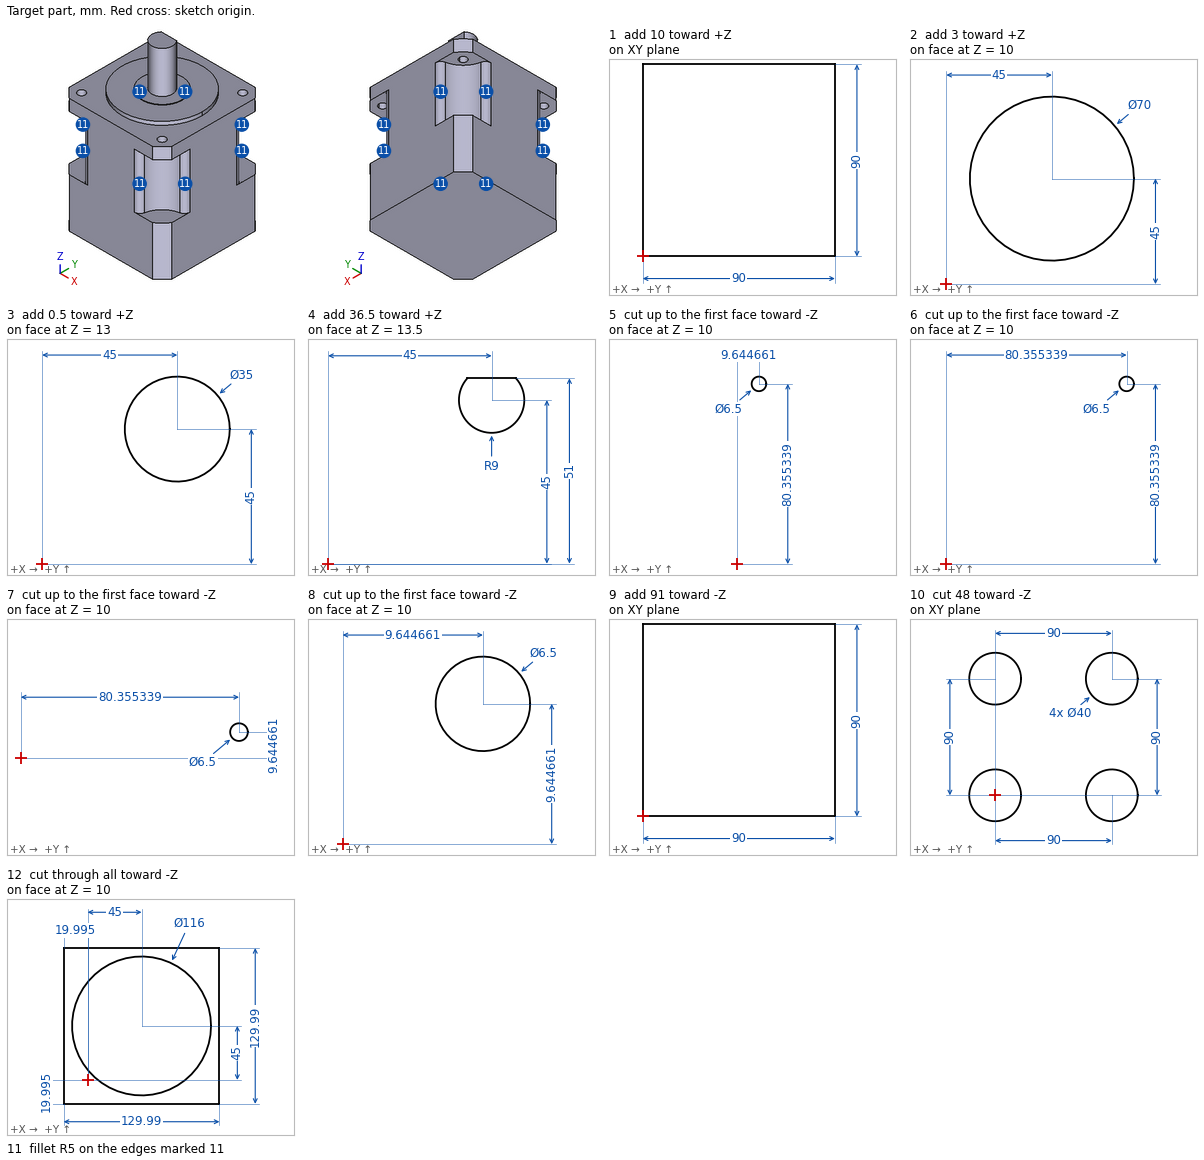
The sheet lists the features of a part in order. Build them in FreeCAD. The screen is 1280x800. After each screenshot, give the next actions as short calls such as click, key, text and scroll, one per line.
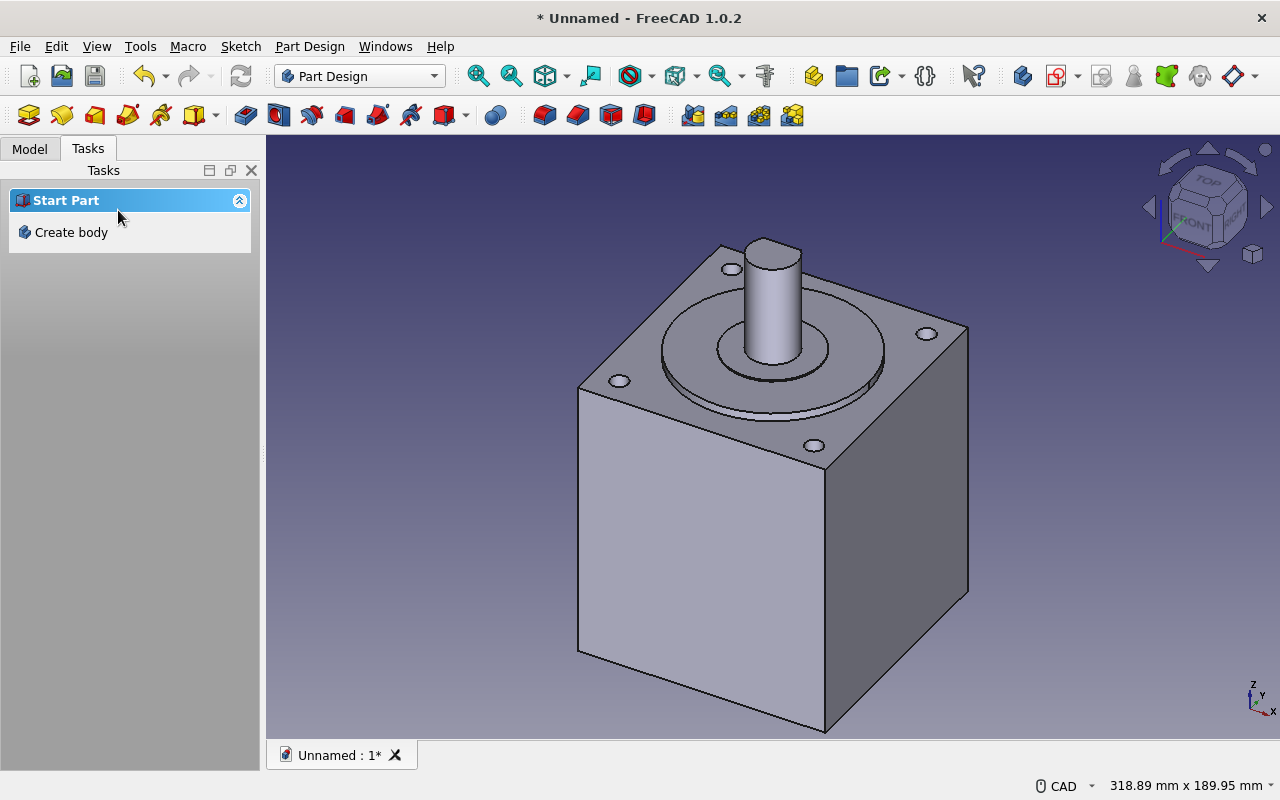
click(1056, 76)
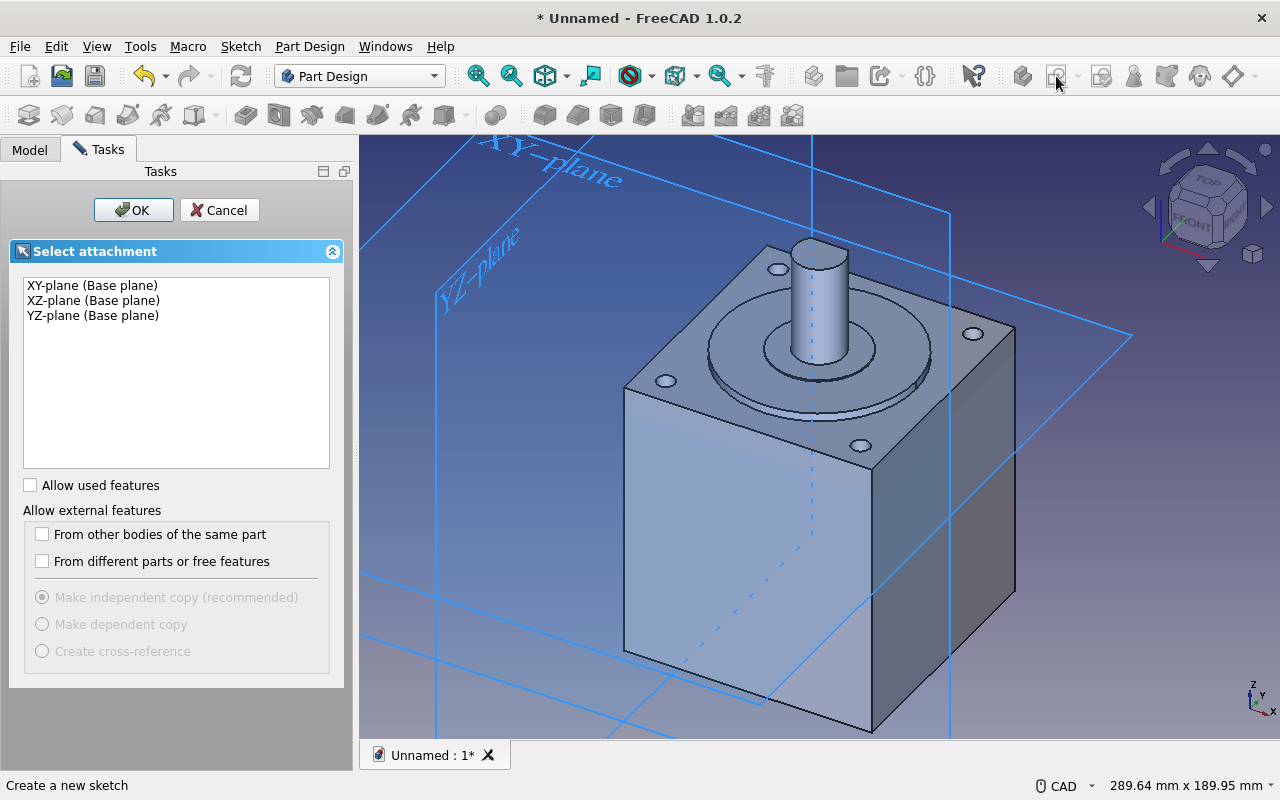
click(84, 286)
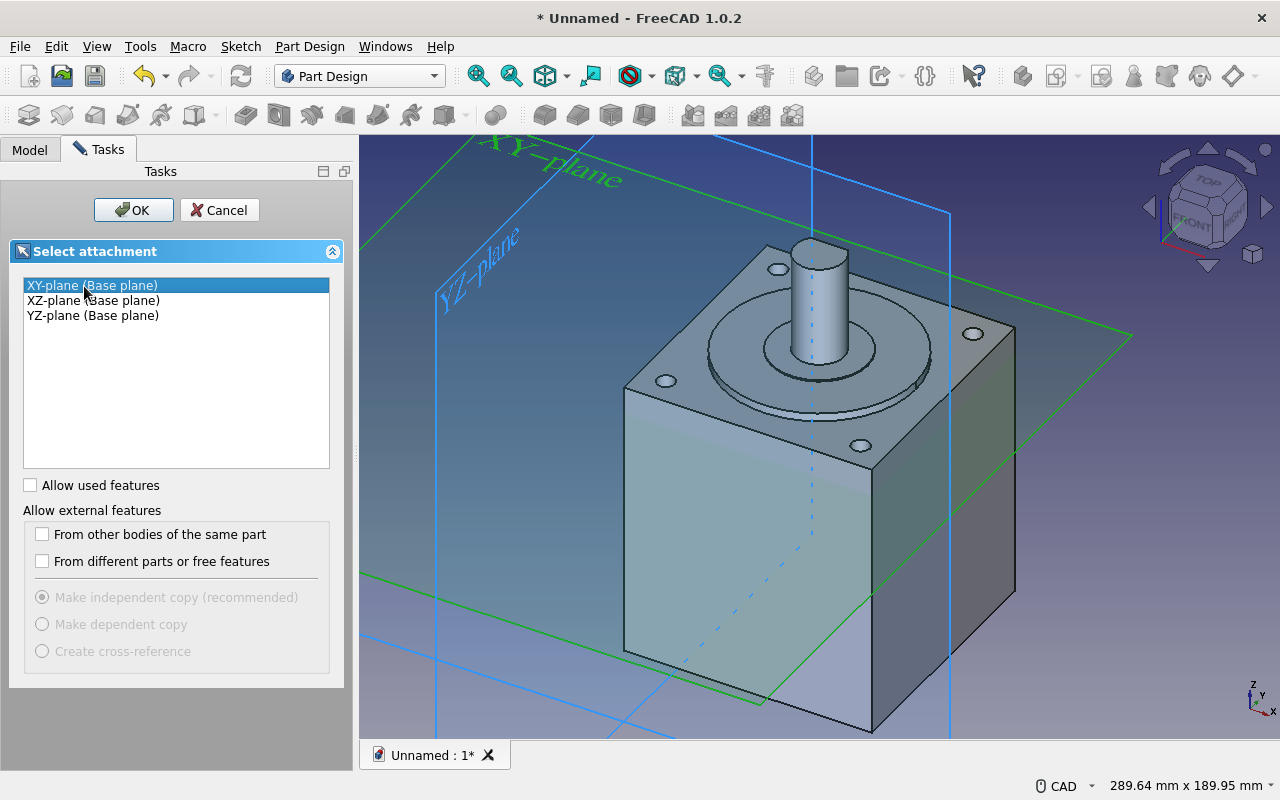
click(134, 210)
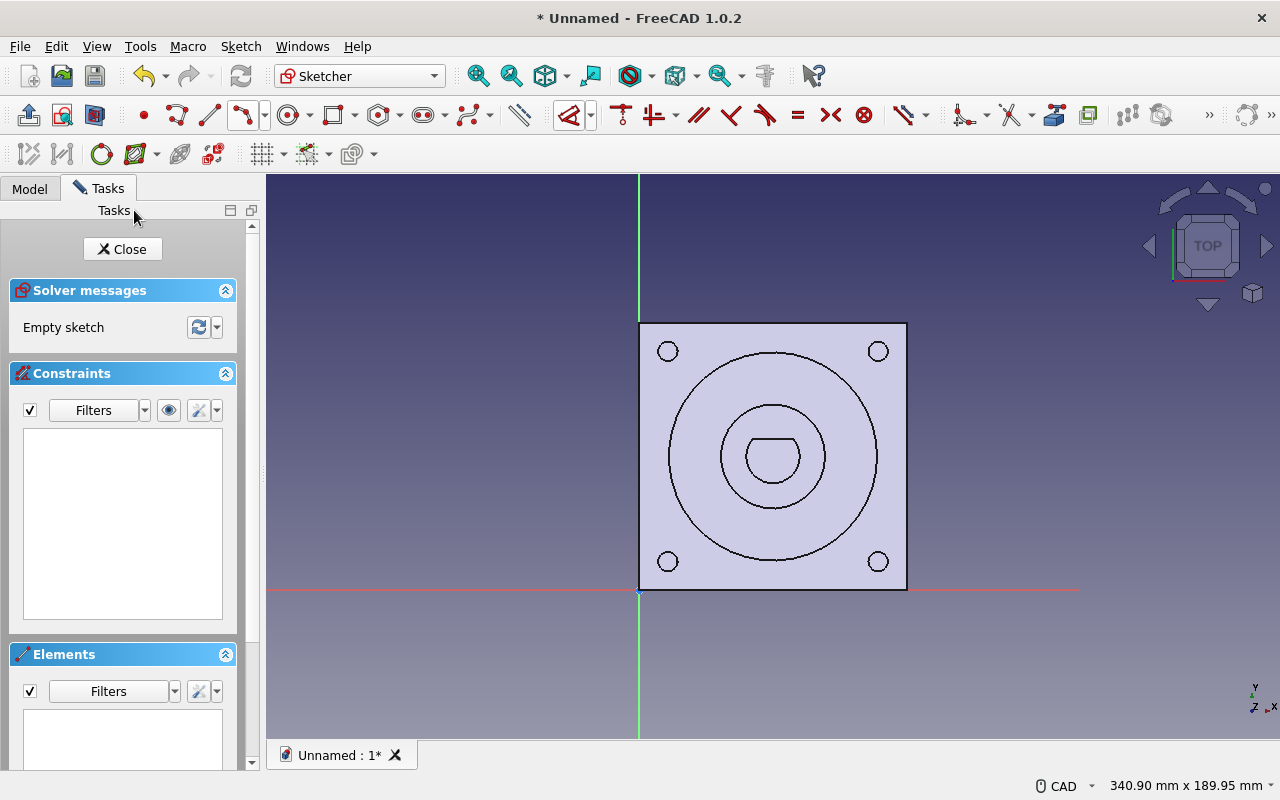
key(q)
key(s)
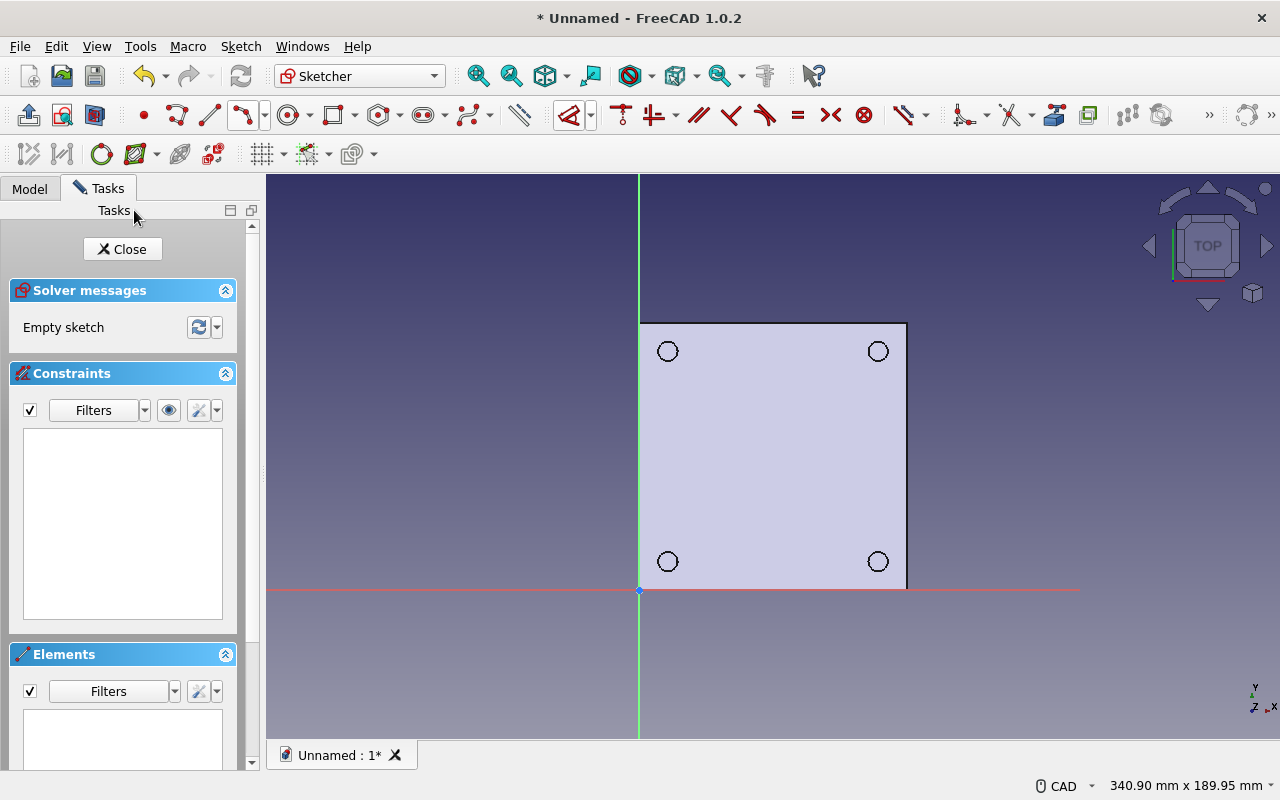
key(g)
key(c)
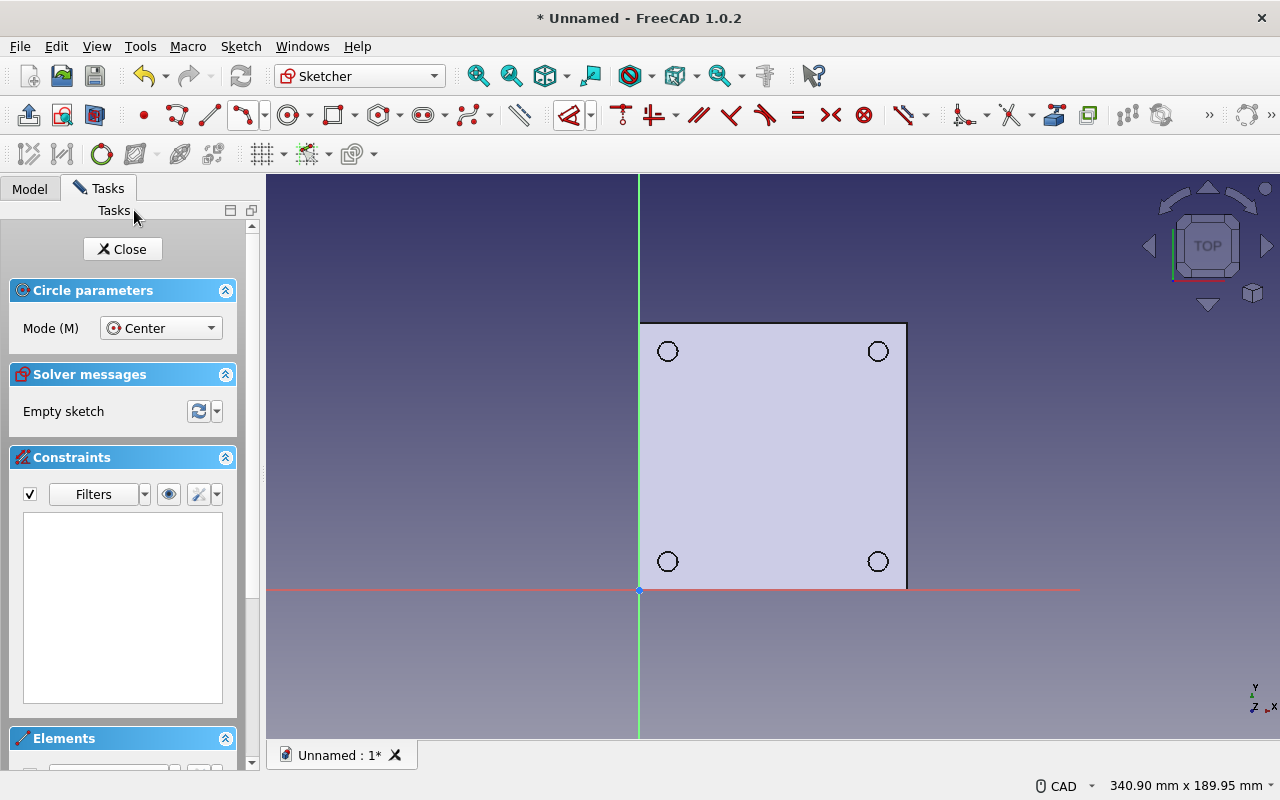
click(907, 323)
move(949, 281)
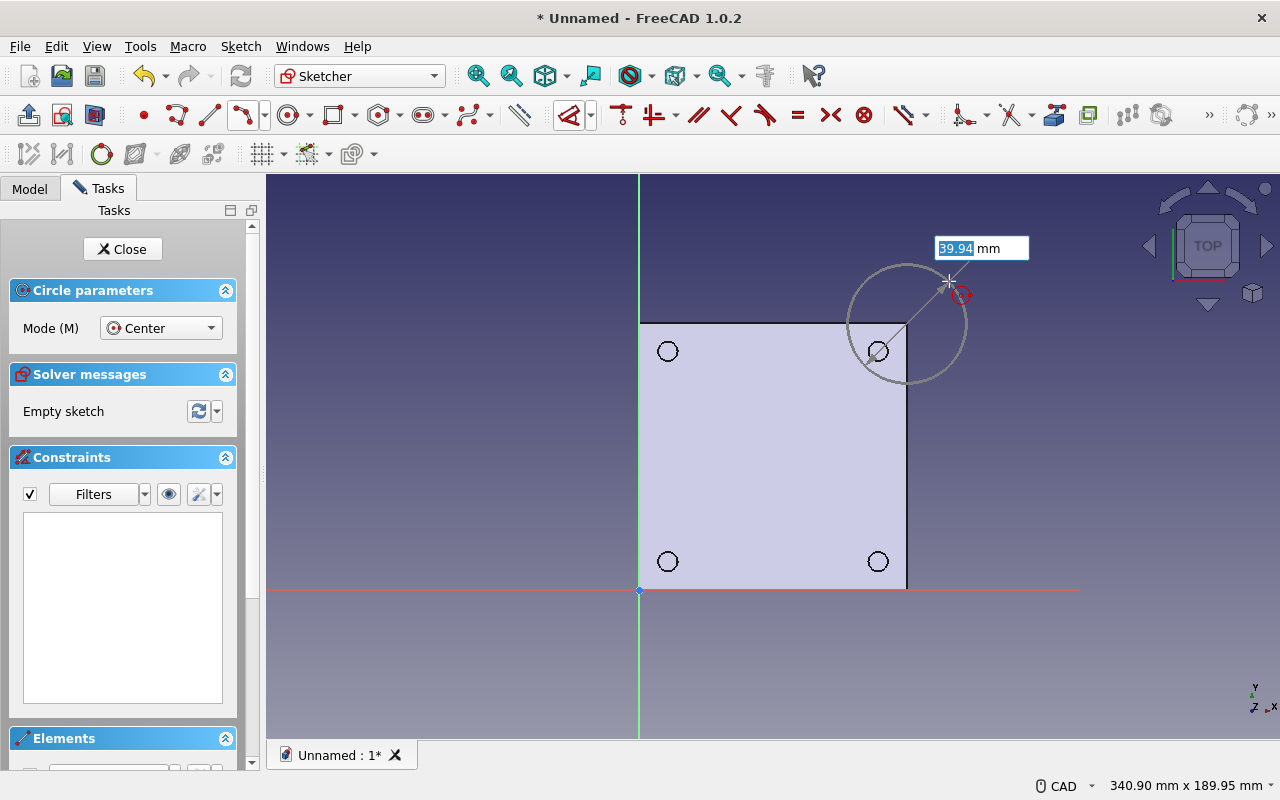
text(40)
key(Return)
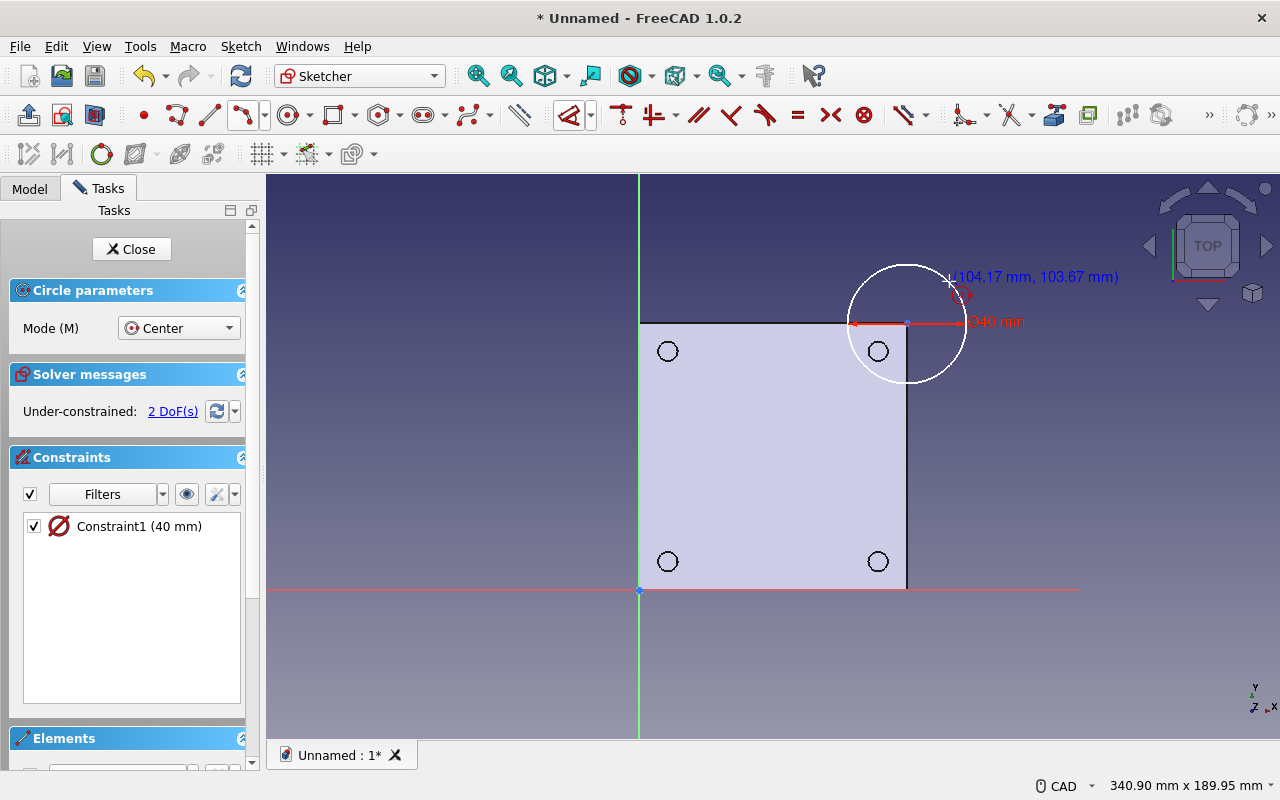
click(907, 590)
move(949, 548)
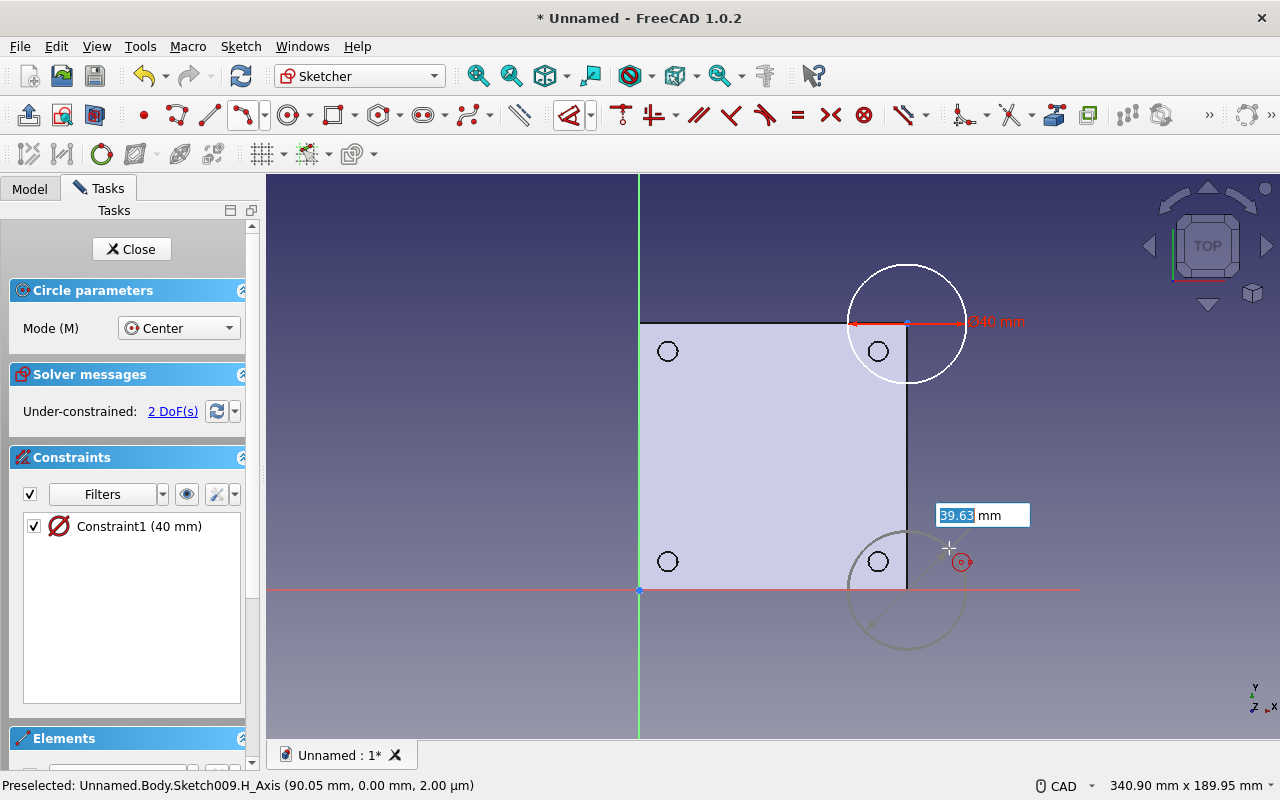
text(40)
key(Return)